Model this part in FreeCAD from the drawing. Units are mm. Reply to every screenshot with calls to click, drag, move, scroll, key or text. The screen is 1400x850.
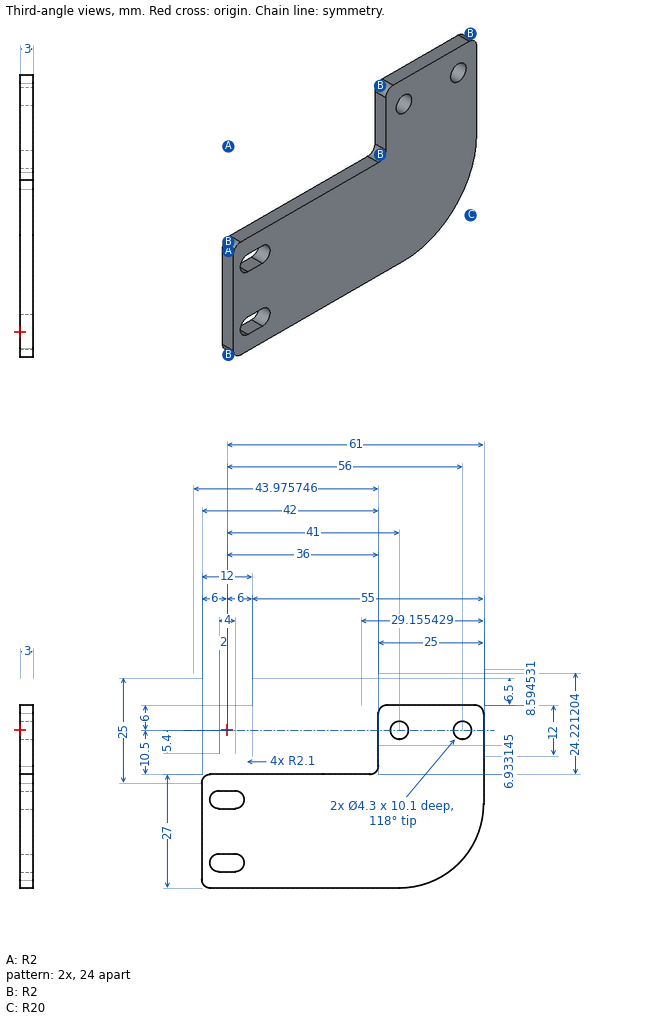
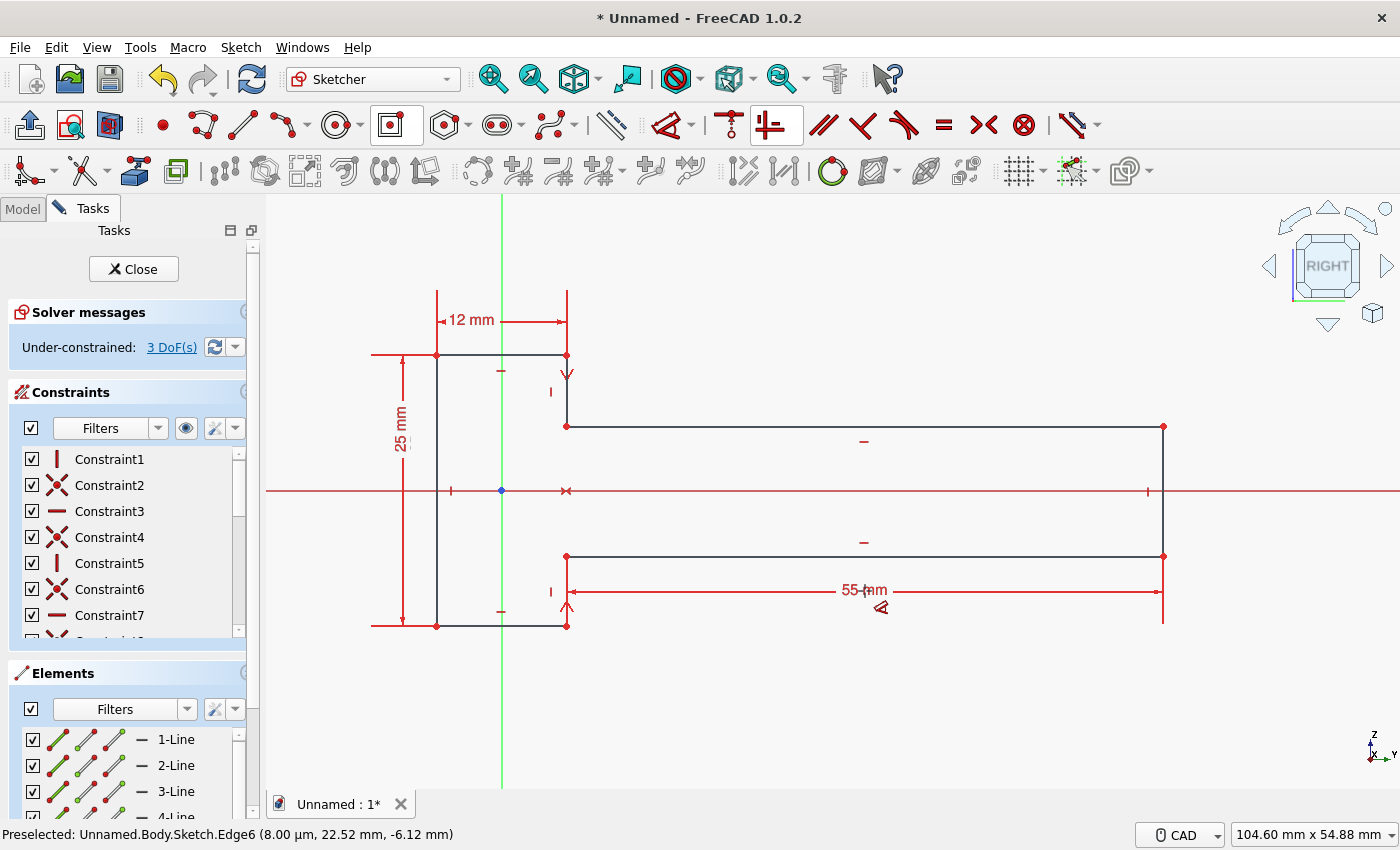
click(1163, 518)
click(1197, 462)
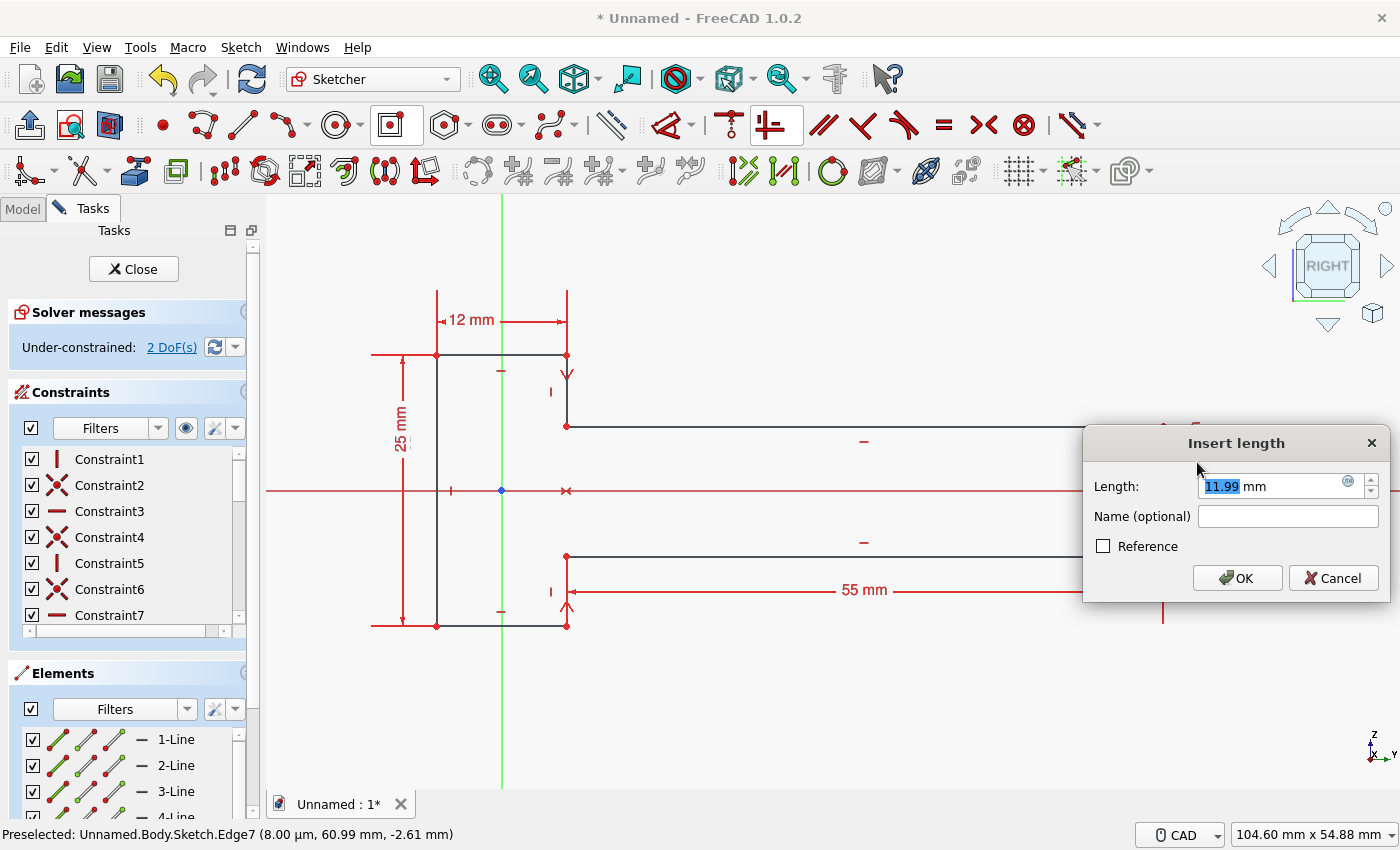
text(12)
key(Return)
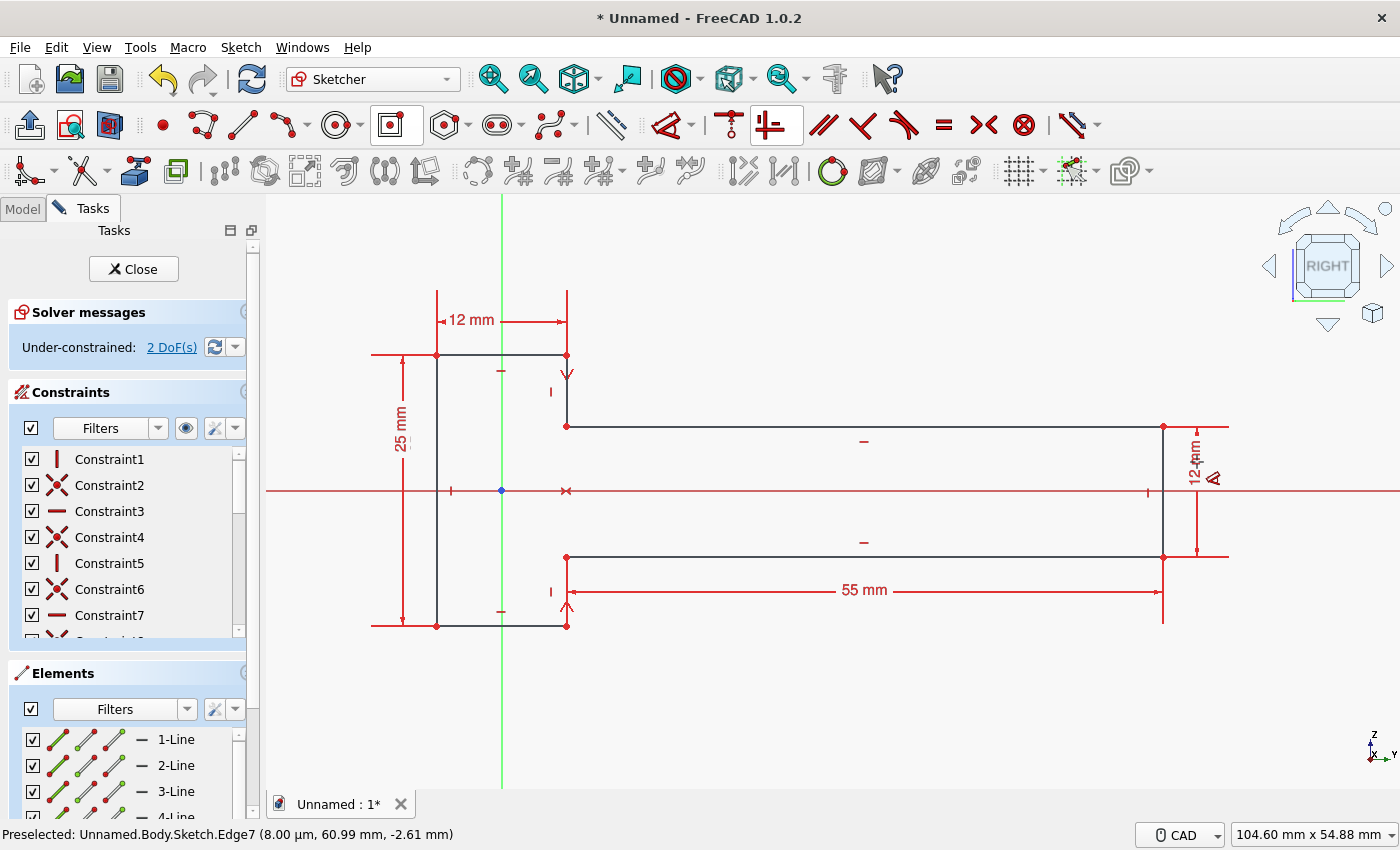
click(567, 427)
click(534, 393)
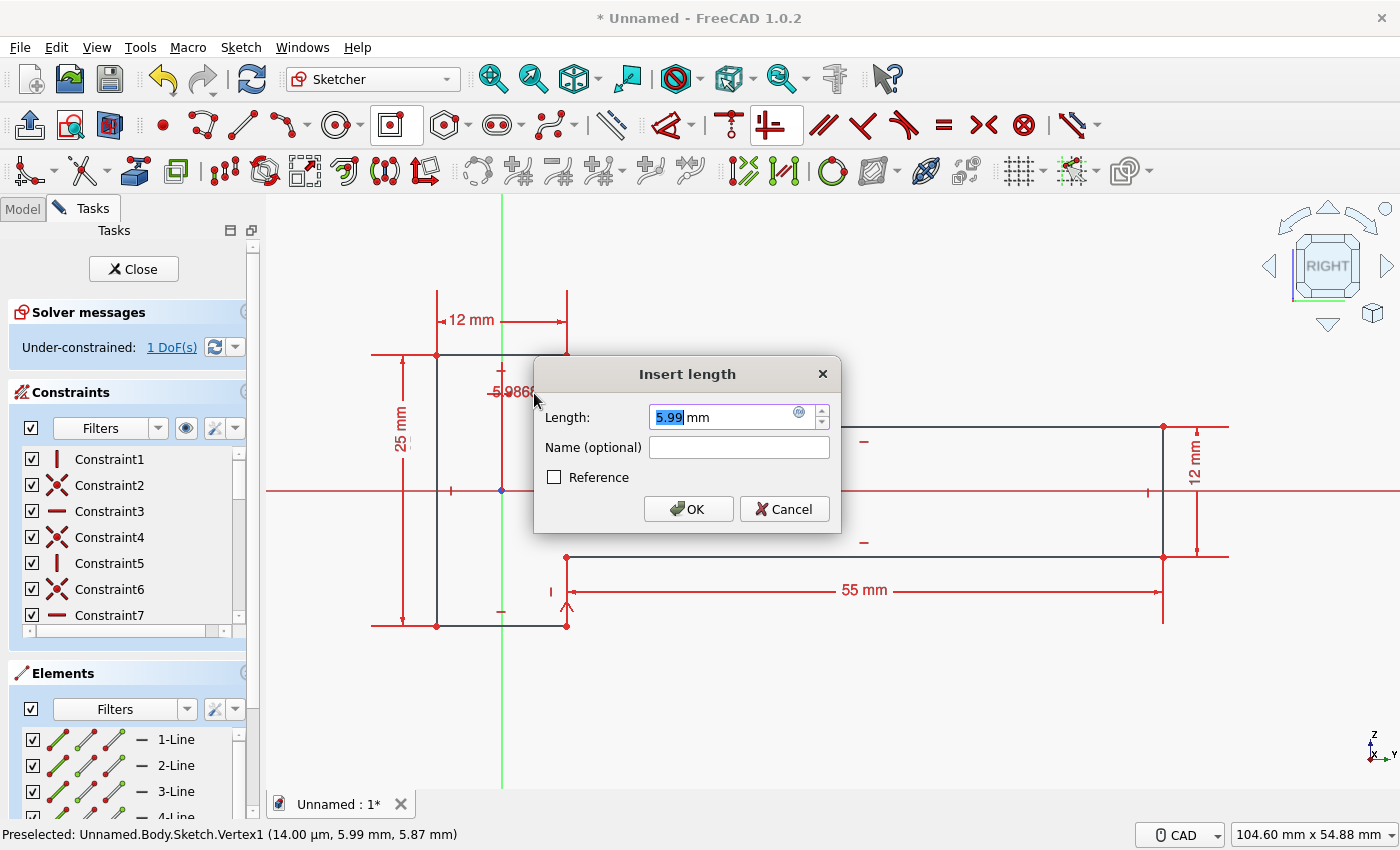
text(6)
key(Return)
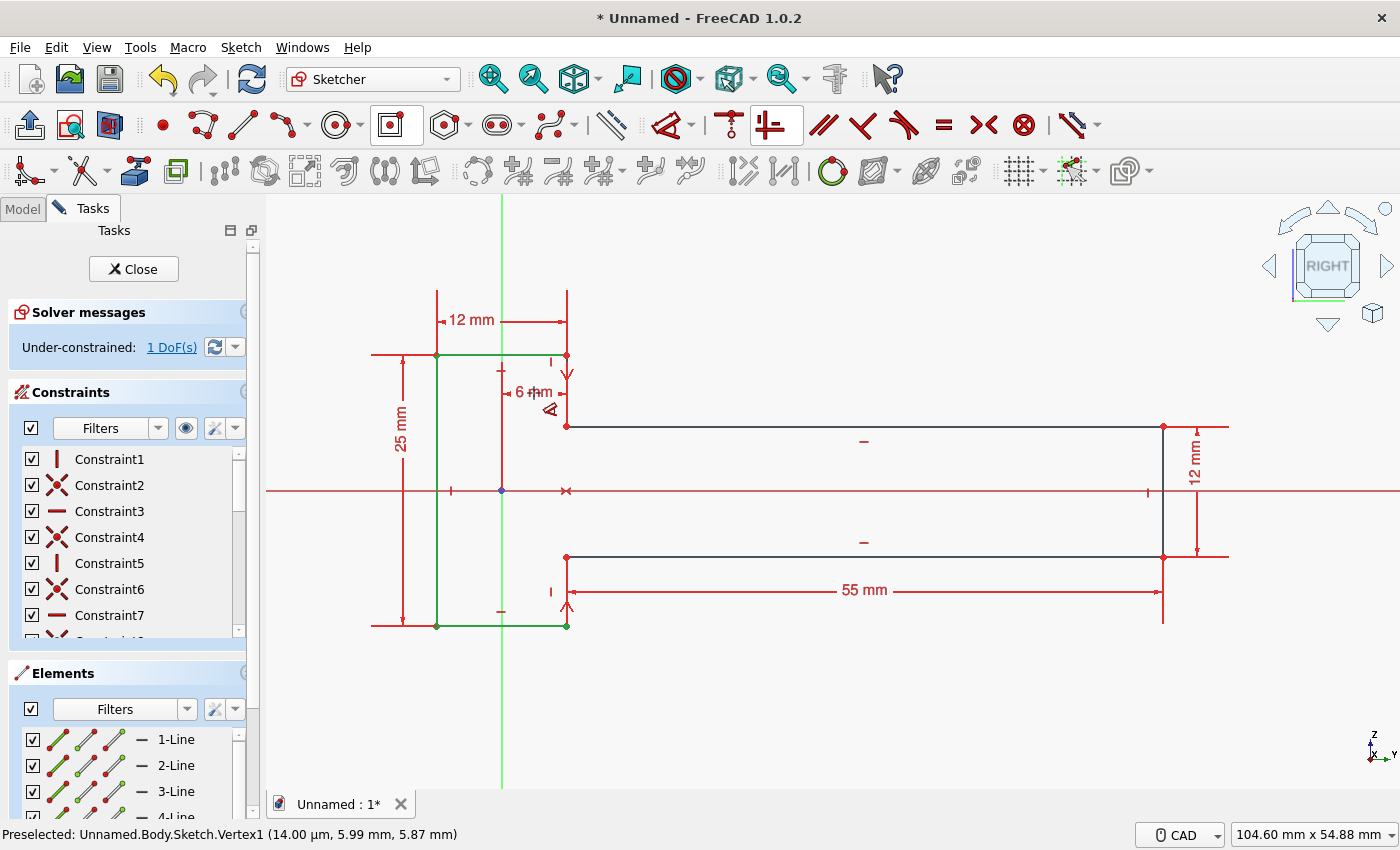
click(567, 427)
click(468, 459)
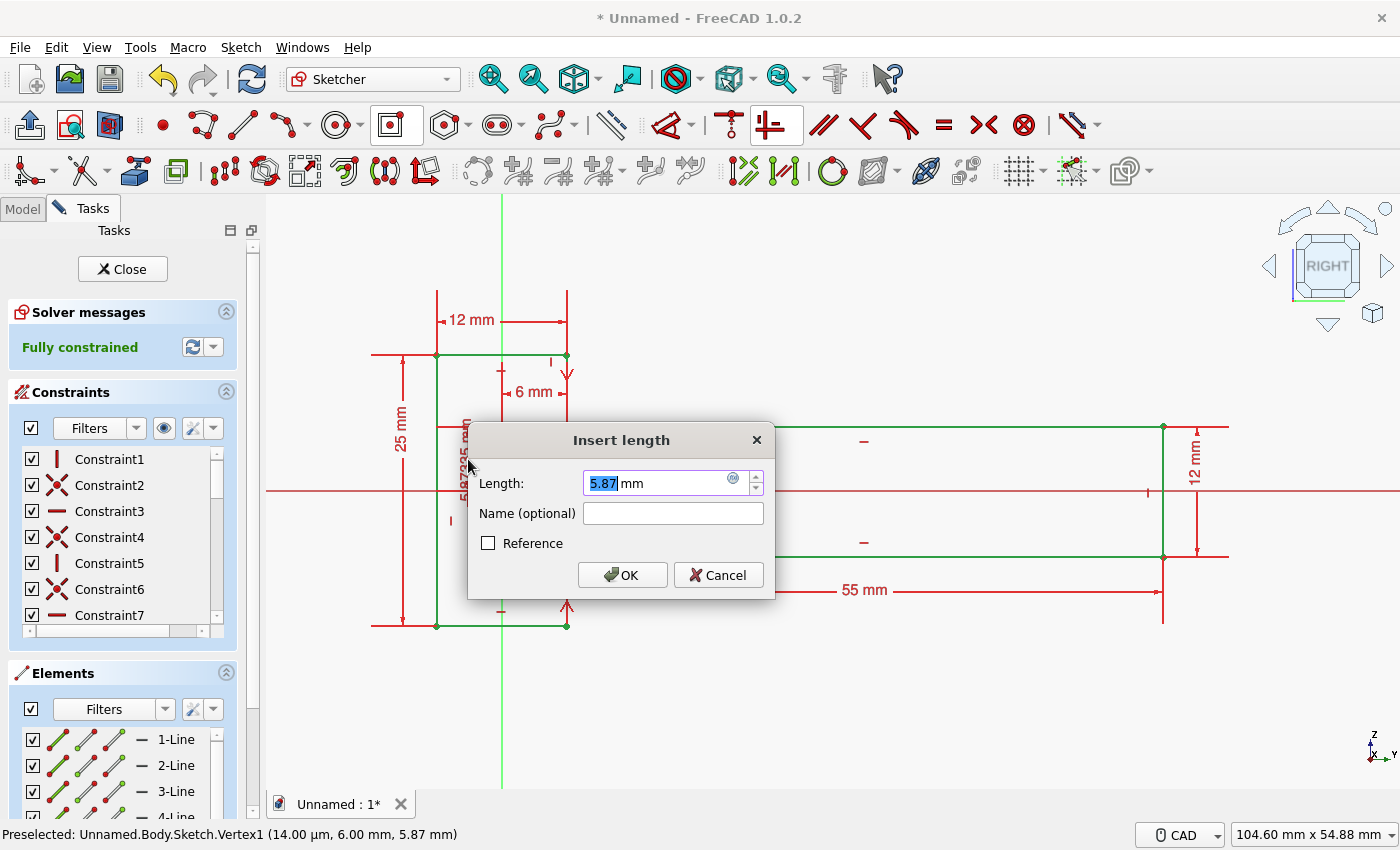
text(6)
key(Return)
key(Escape)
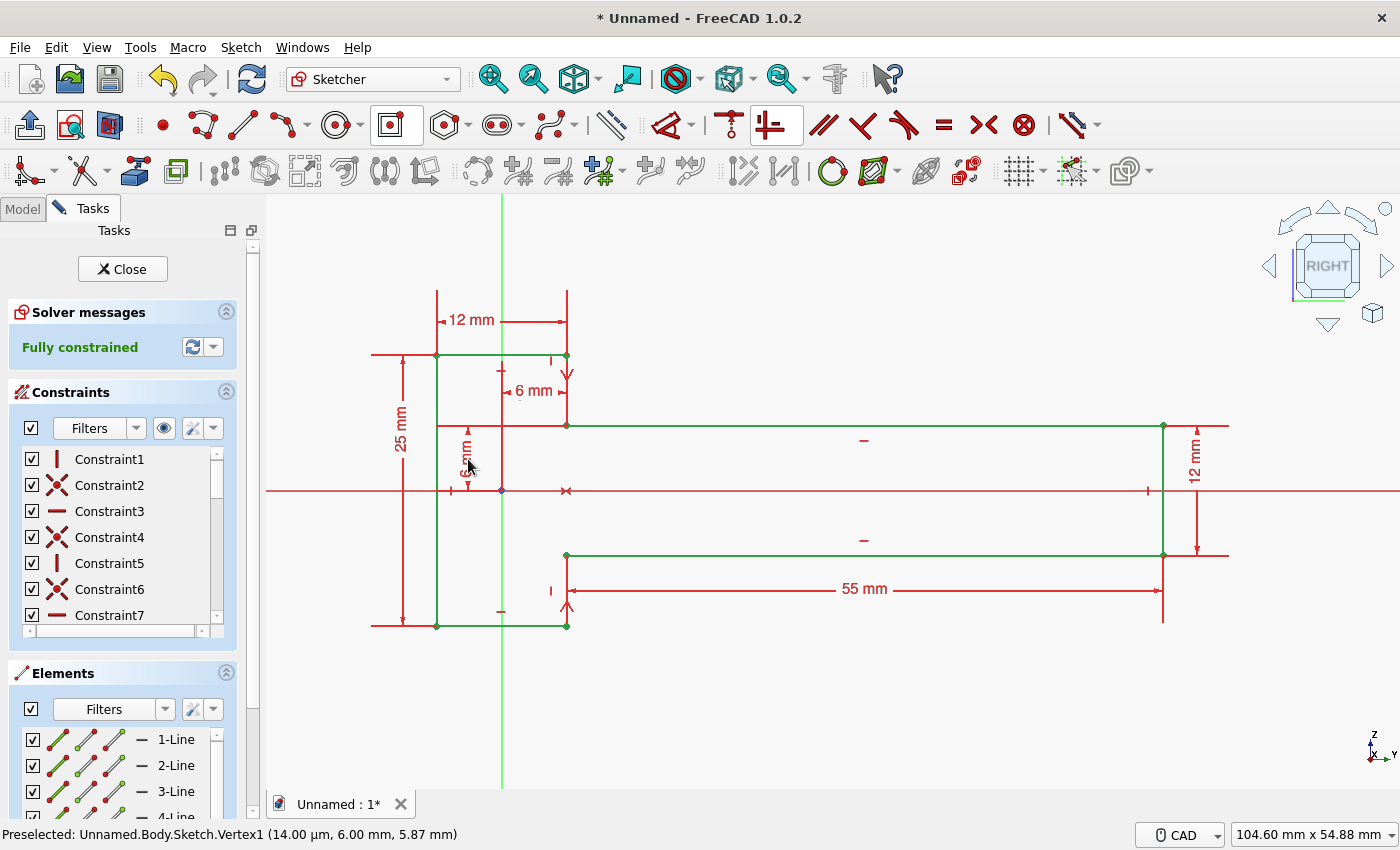
click(123, 269)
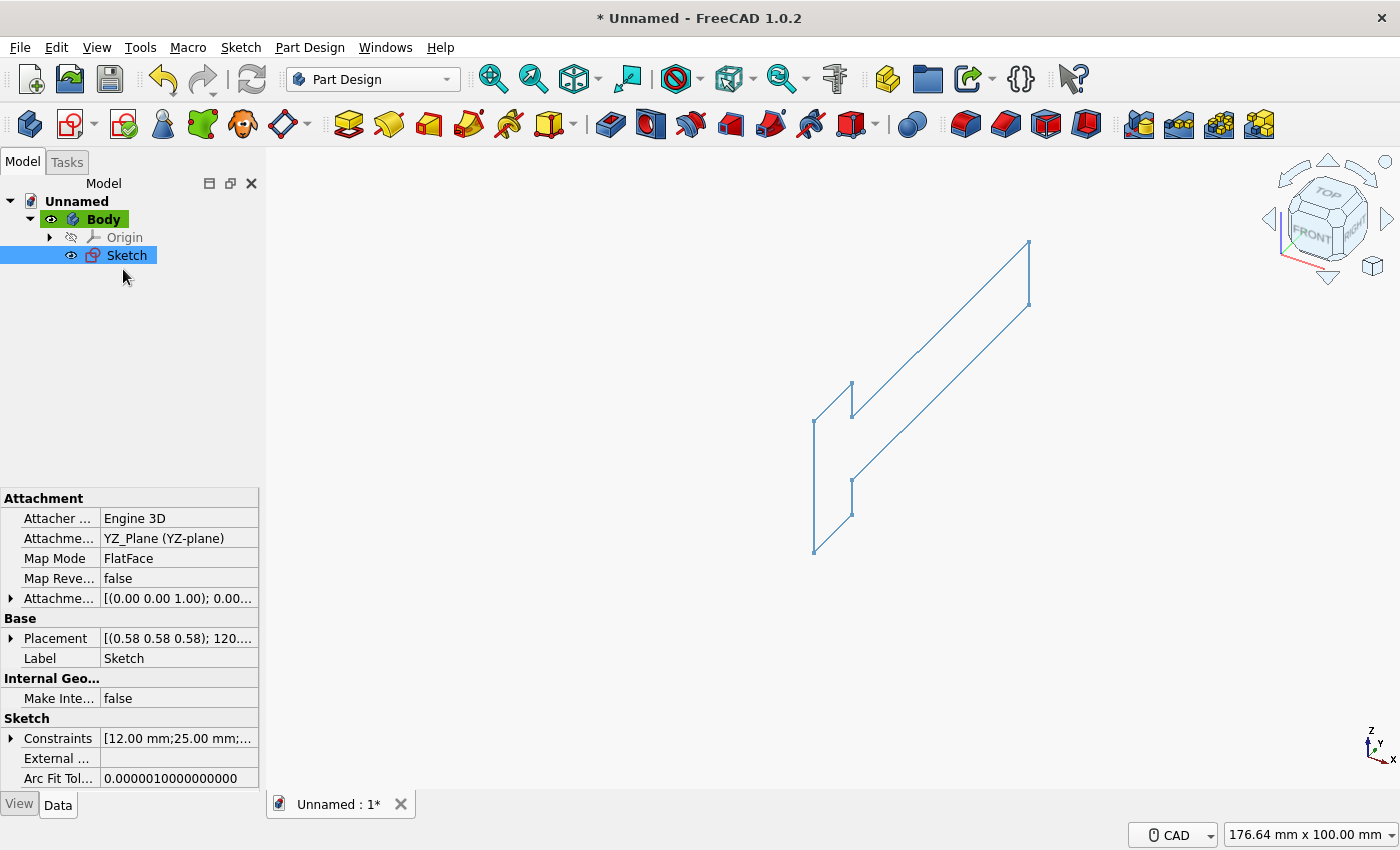
click(350, 124)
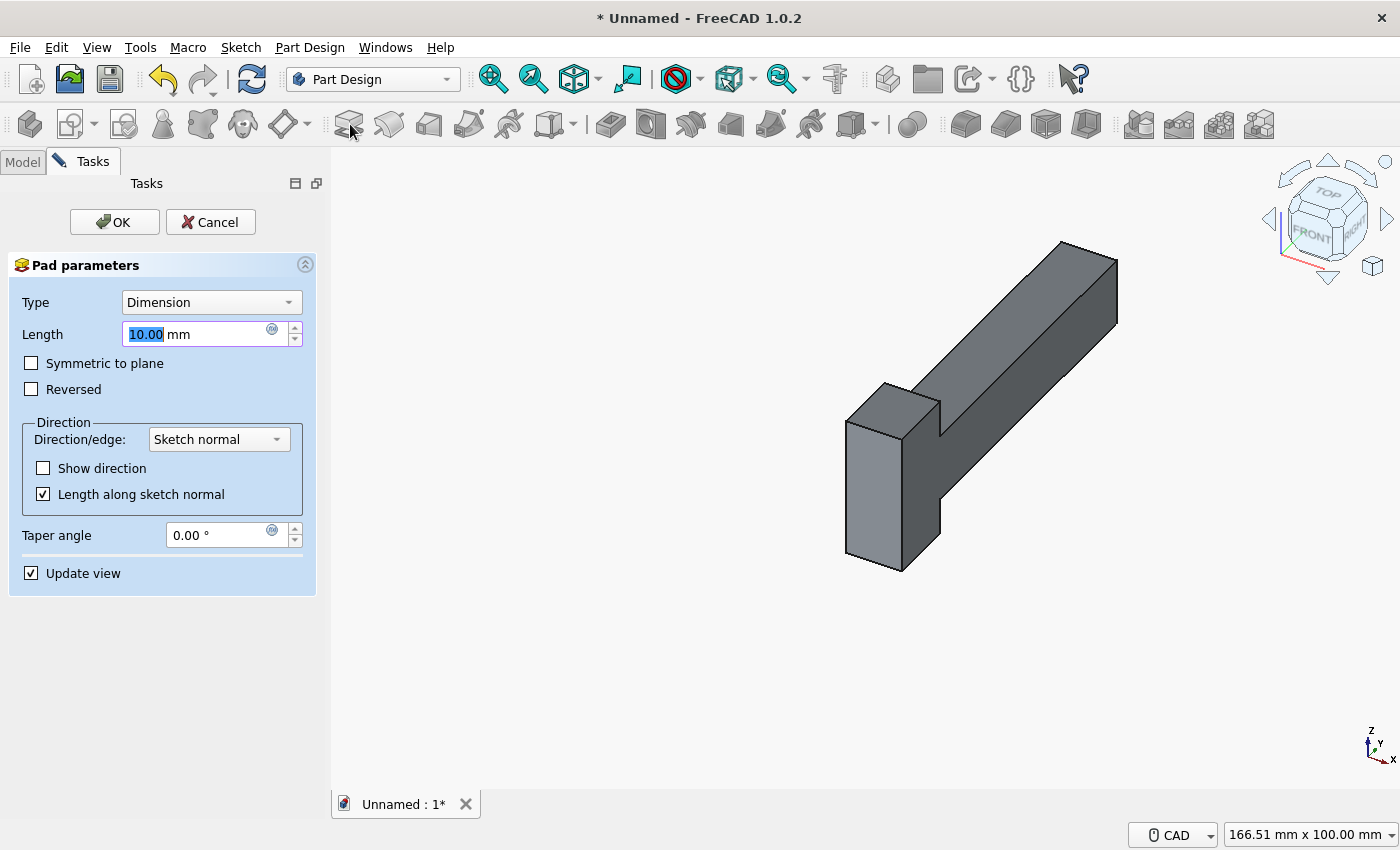
text(3)
key(Tab)